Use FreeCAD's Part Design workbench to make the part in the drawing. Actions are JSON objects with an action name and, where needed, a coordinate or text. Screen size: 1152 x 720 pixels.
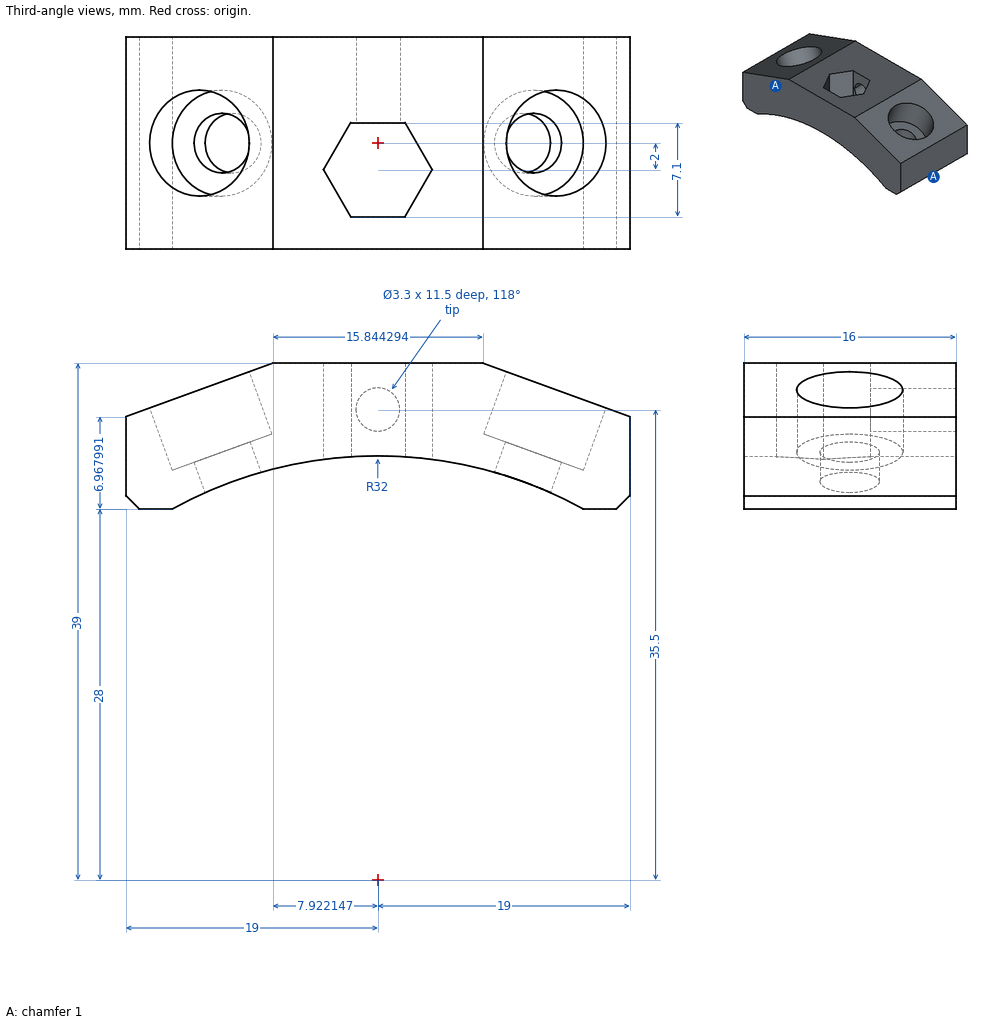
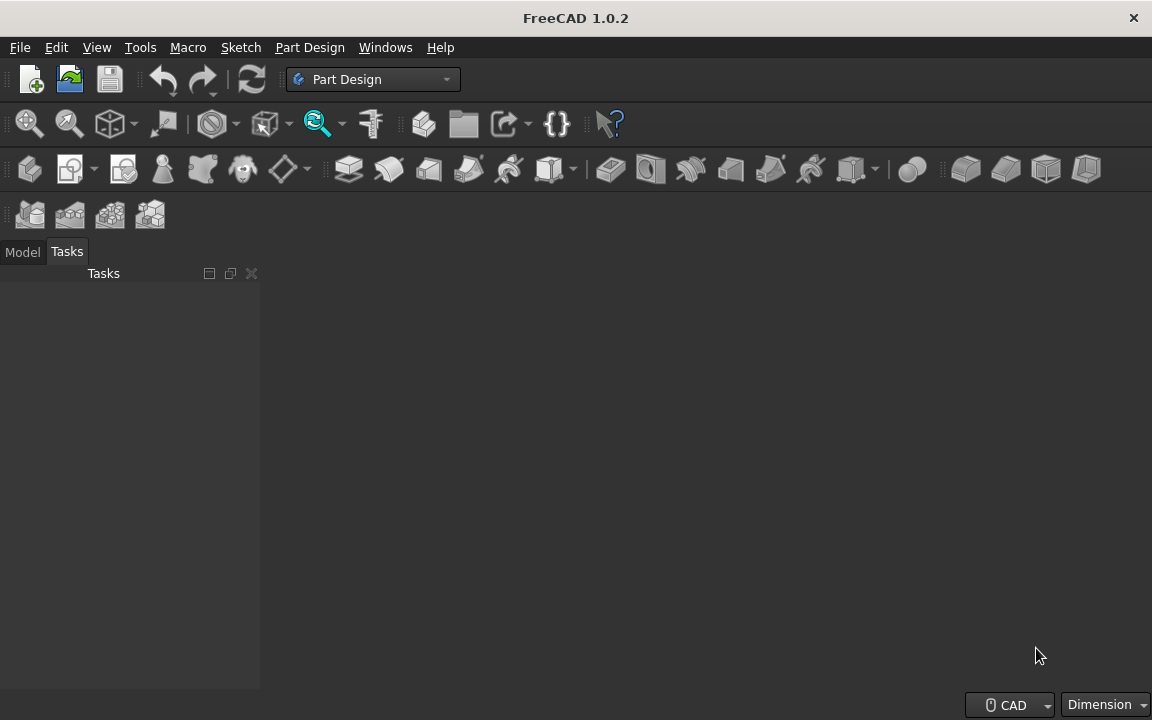
{"action": "key", "text": "ctrl+n"}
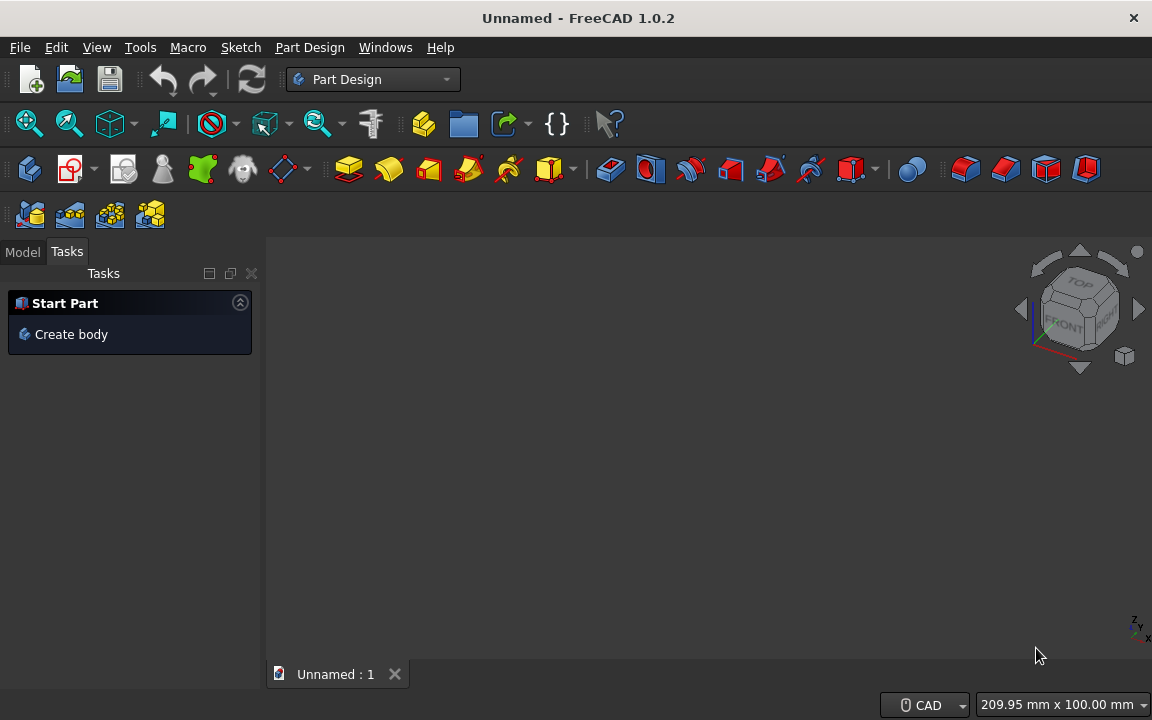
{"action": "left_click", "coordinate": [70, 170]}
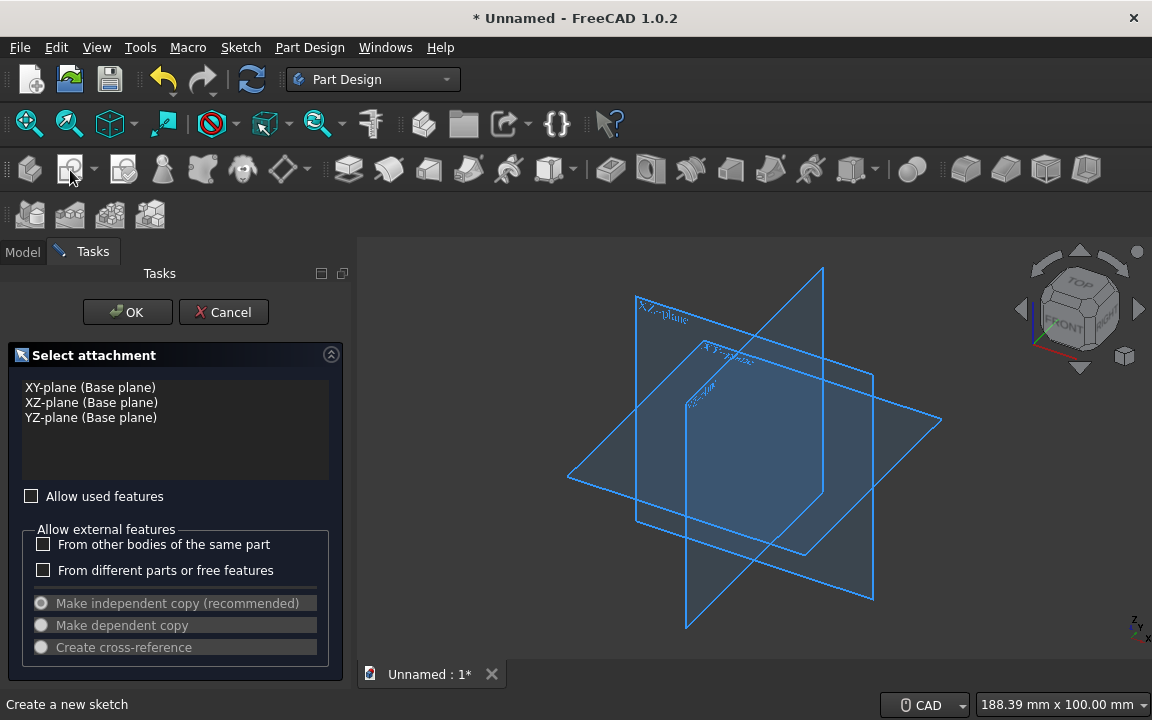
{"action": "left_click", "coordinate": [82, 402]}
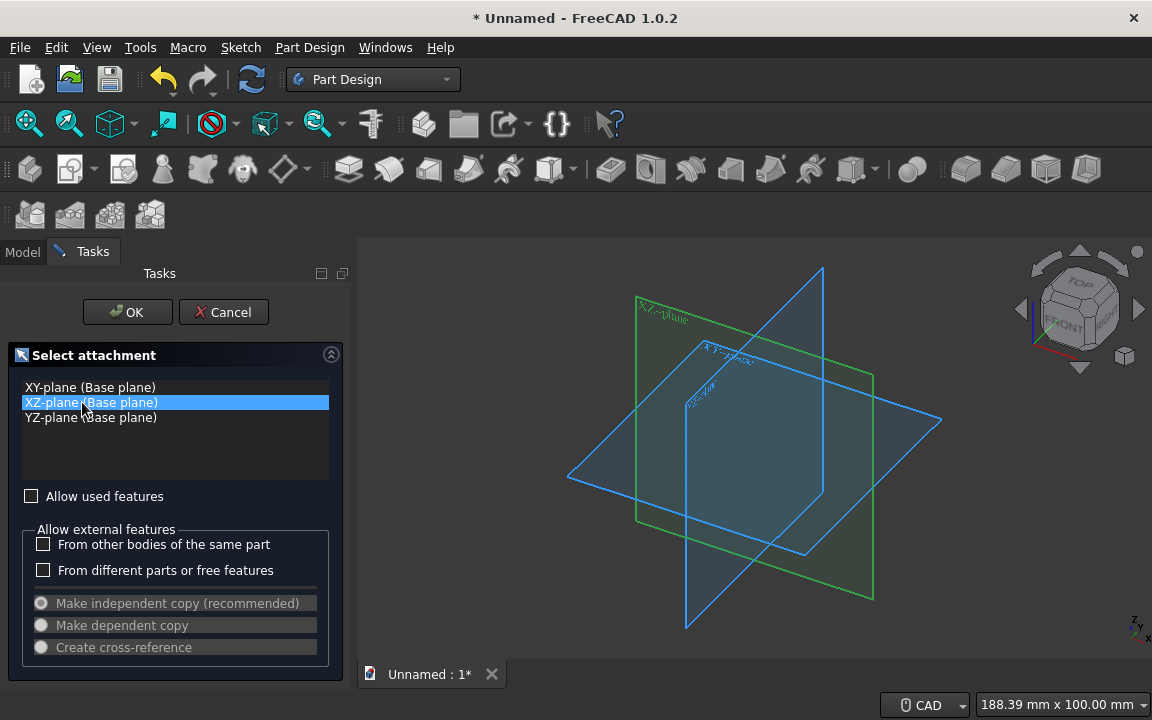
{"action": "left_click", "coordinate": [128, 312]}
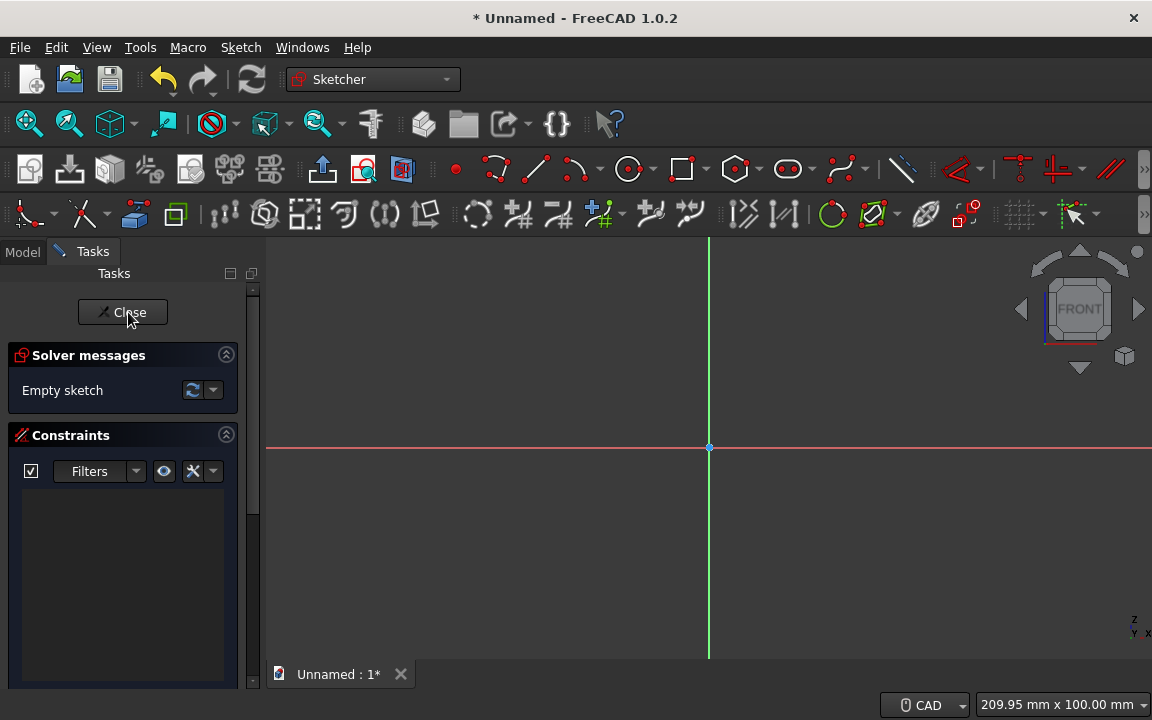
{"action": "scroll", "coordinate": [848, 265], "scroll_direction": "up", "scroll_amount": 2}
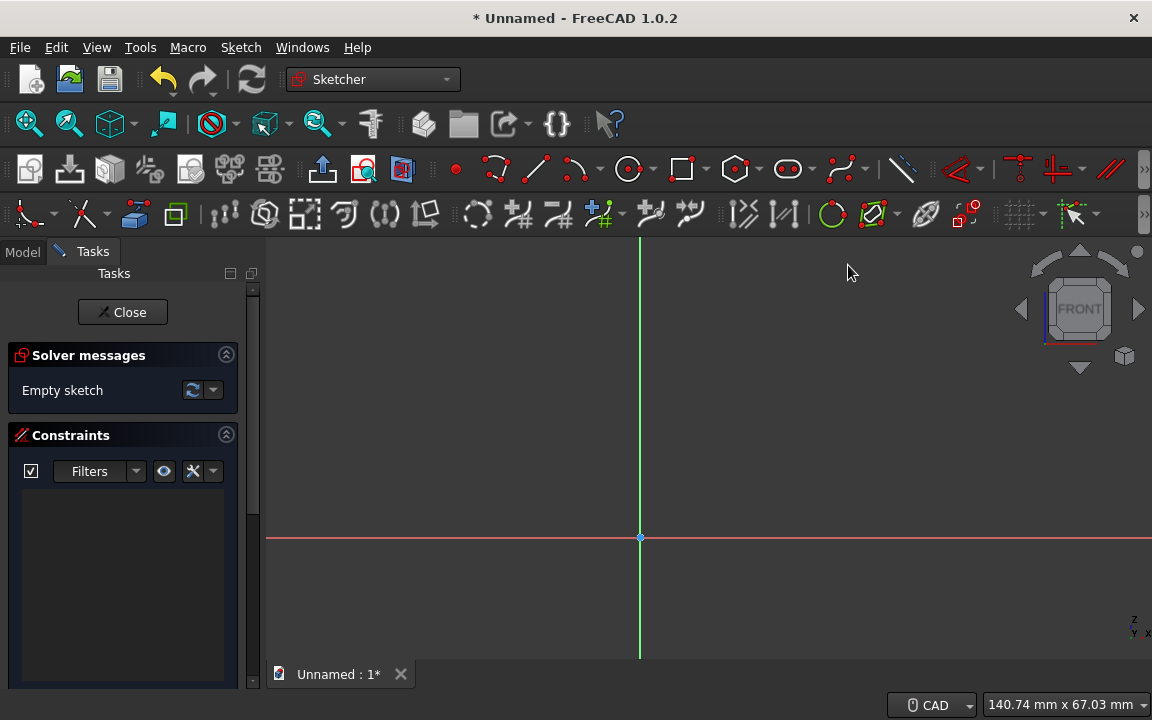
{"action": "key", "text": "g m"}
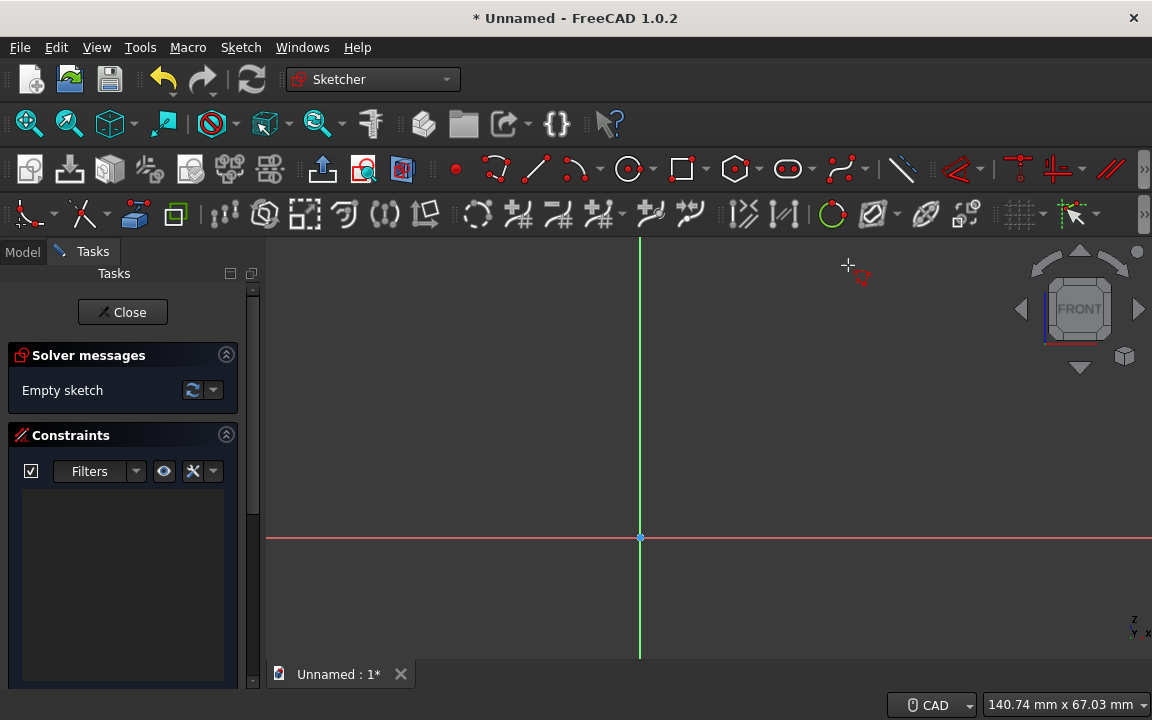
{"action": "left_click", "coordinate": [543, 362]}
{"action": "left_click", "coordinate": [521, 362]}
{"action": "left_click", "coordinate": [521, 318]}
{"action": "left_click", "coordinate": [590, 292]}
{"action": "left_click", "coordinate": [690, 292]}
{"action": "left_click", "coordinate": [760, 318]}
{"action": "left_click", "coordinate": [760, 362]}
{"action": "left_click", "coordinate": [738, 362]}
{"action": "right_click", "coordinate": [738, 362]}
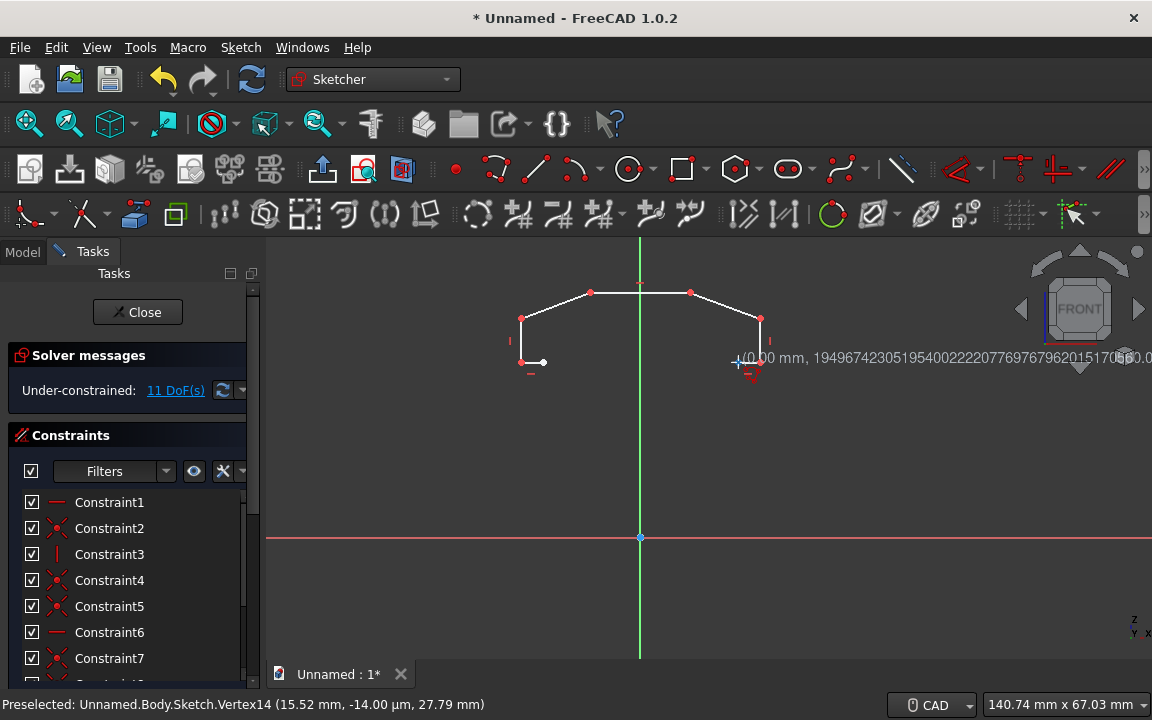
{"action": "key", "text": "g 3 a"}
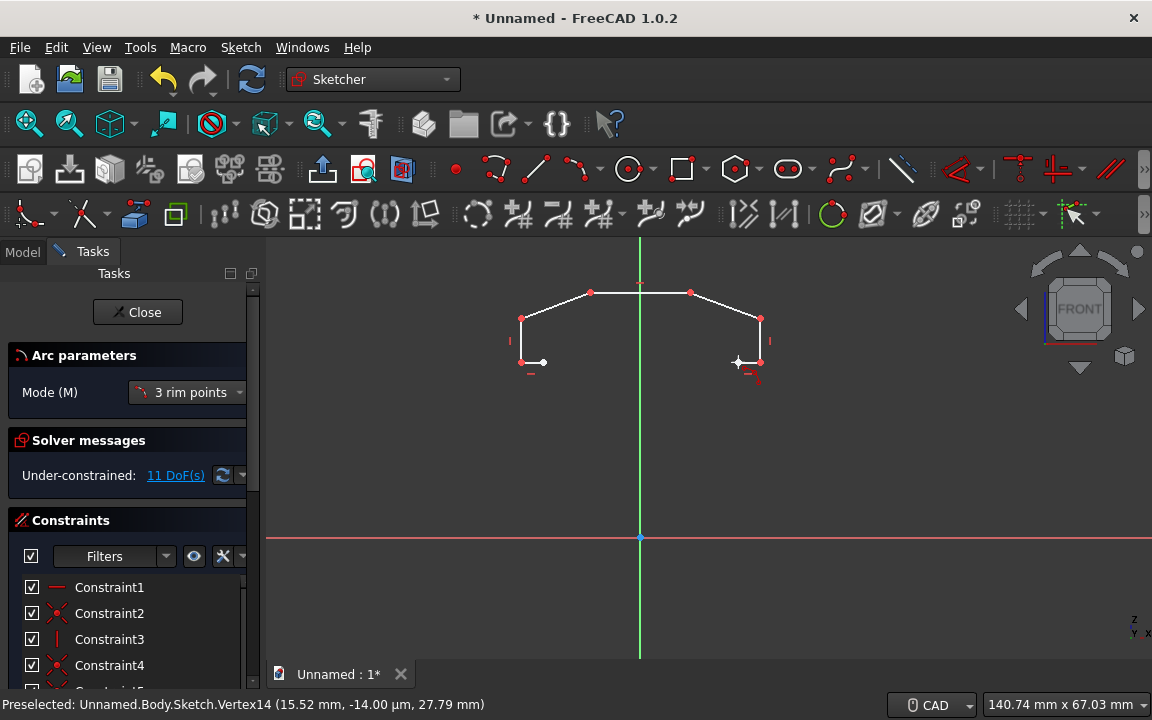
{"action": "scroll", "coordinate": [738, 362], "scroll_direction": "up", "scroll_amount": 2}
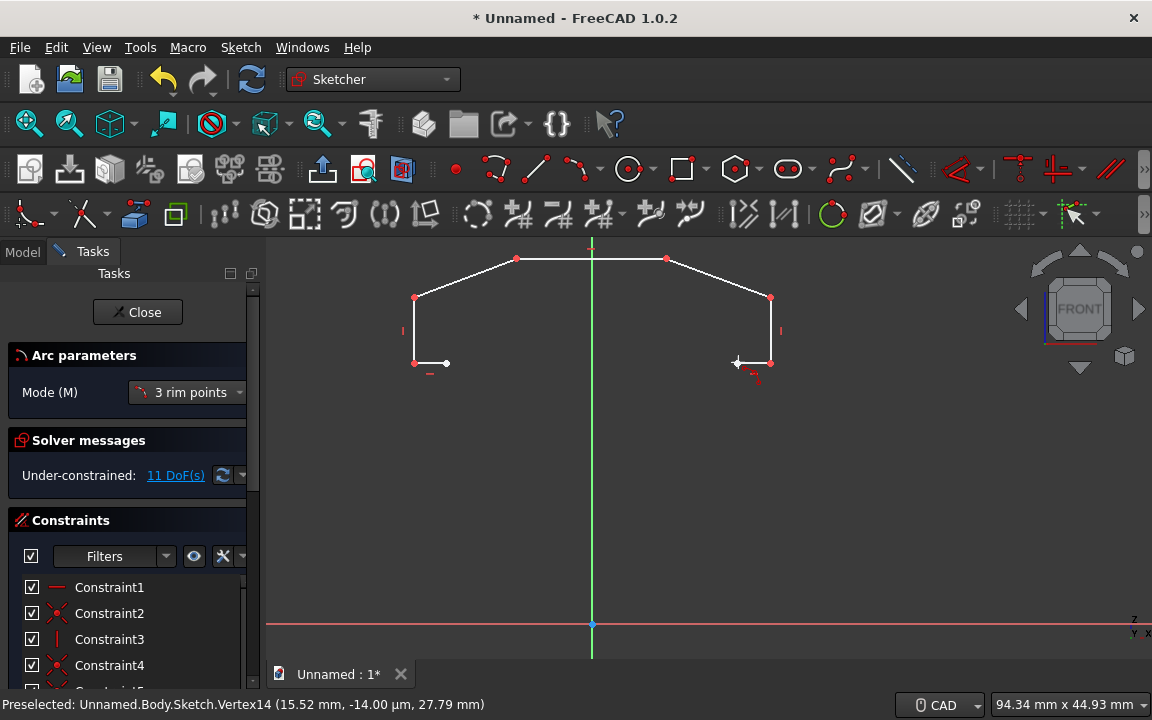
{"action": "left_click", "coordinate": [738, 363]}
{"action": "left_click", "coordinate": [447, 363]}
{"action": "left_click", "coordinate": [622, 325]}
{"action": "key", "text": "Escape"}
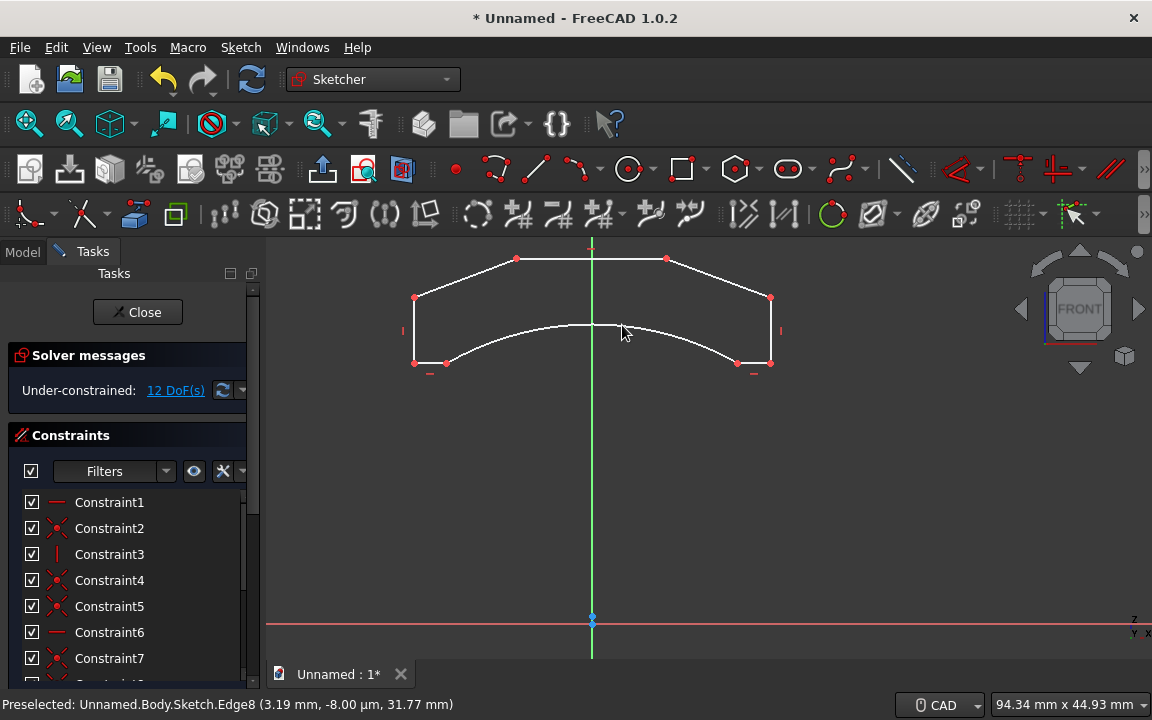
{"action": "left_click_drag", "start_coordinate": [582, 606], "coordinate": [602, 634]}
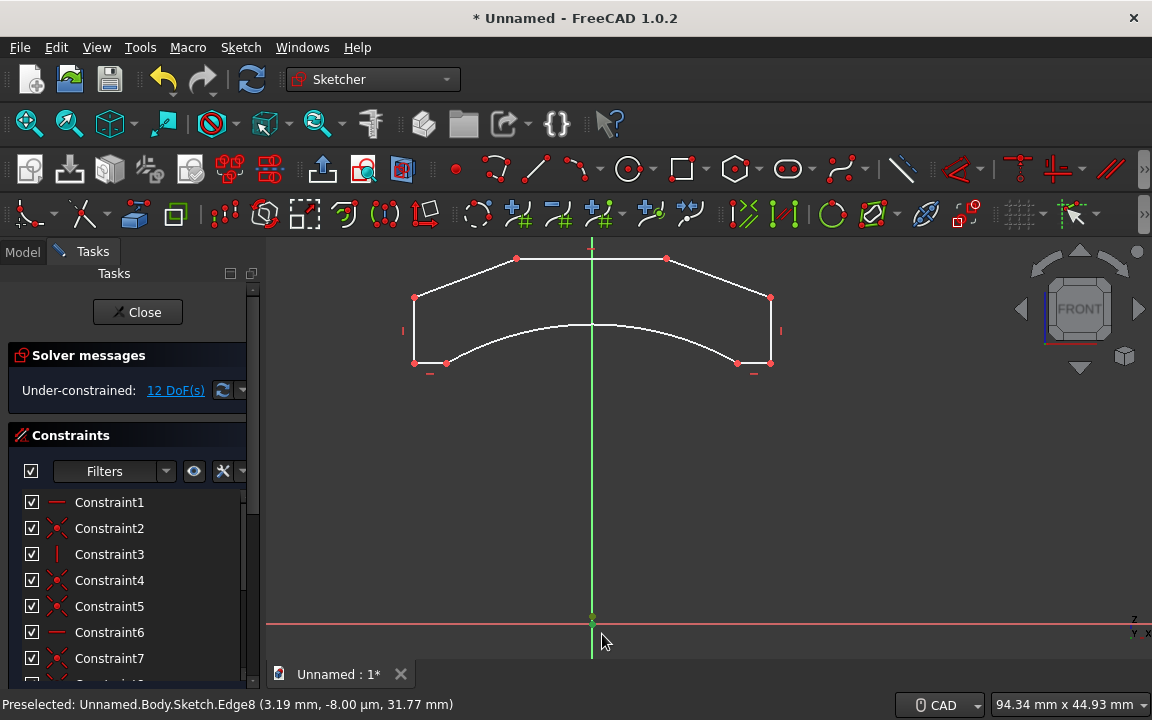
{"action": "key", "text": "c"}